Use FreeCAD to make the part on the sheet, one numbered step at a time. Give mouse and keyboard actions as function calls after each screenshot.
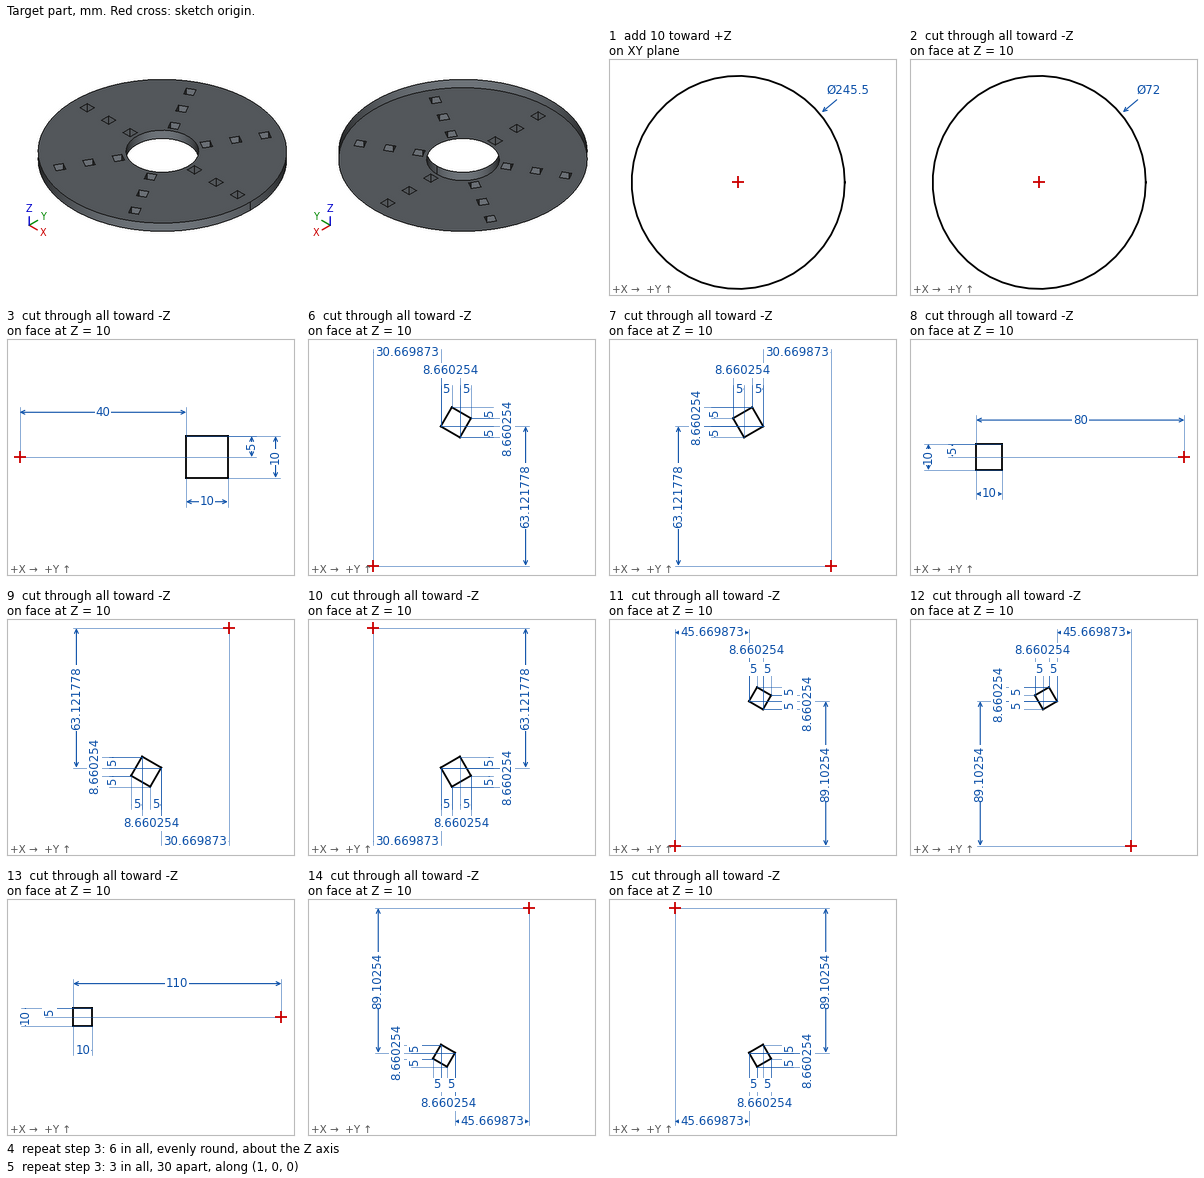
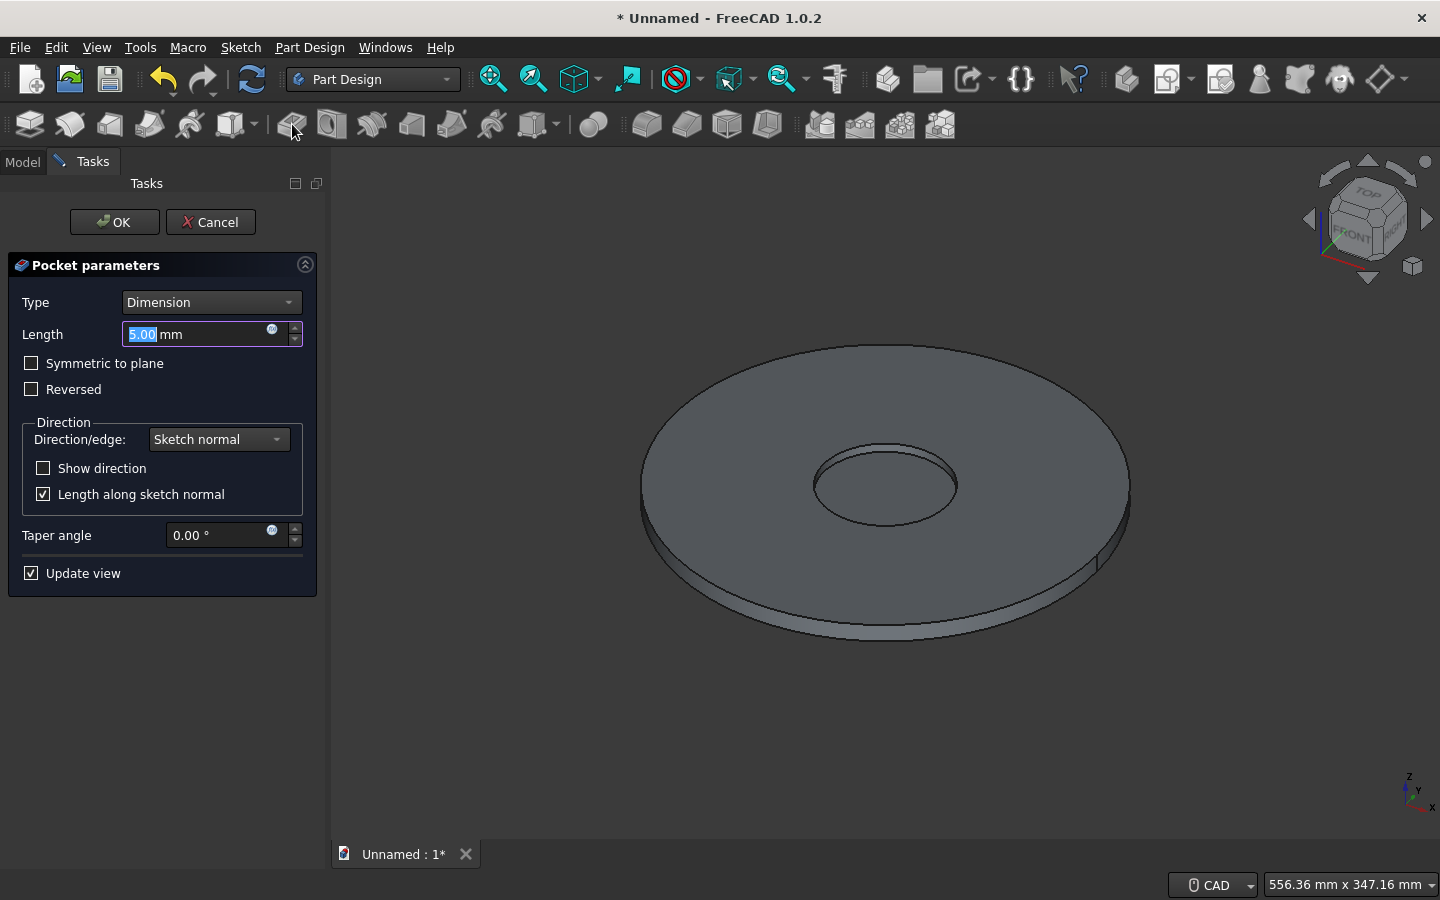
click(212, 302)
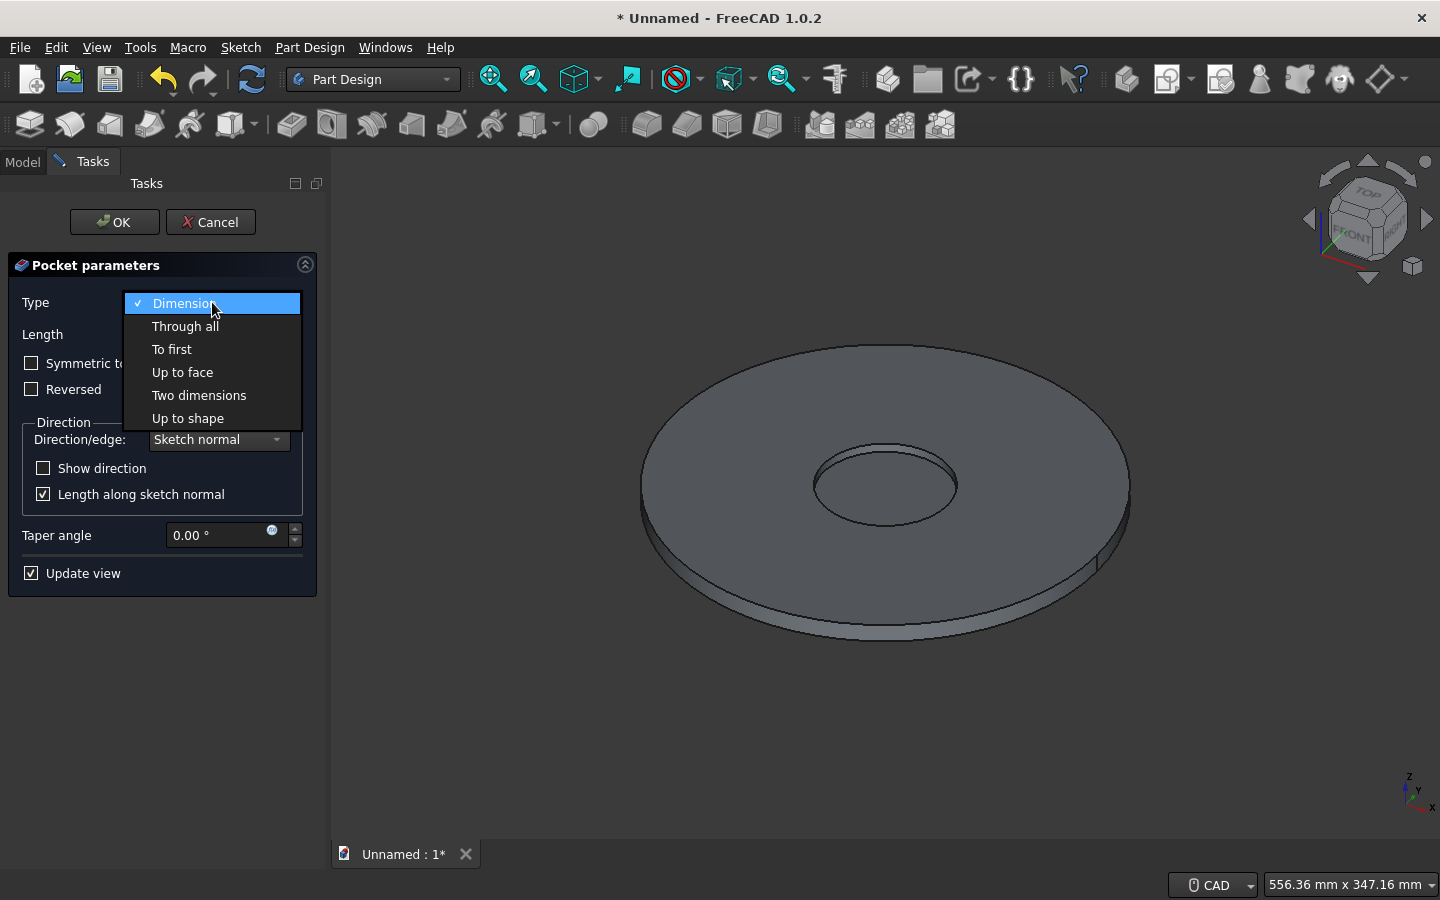
click(212, 326)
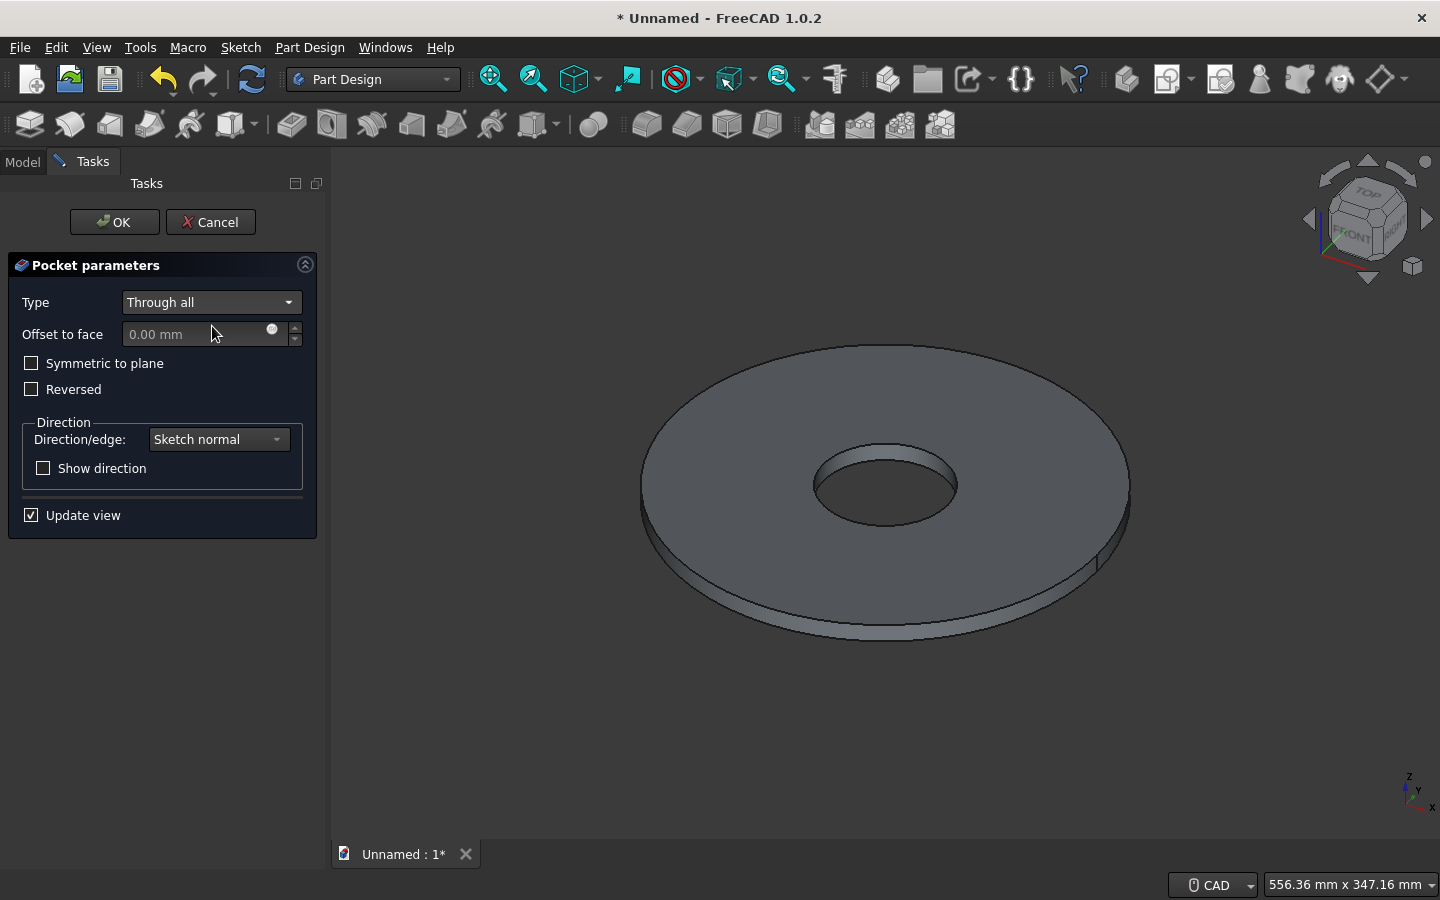
click(115, 222)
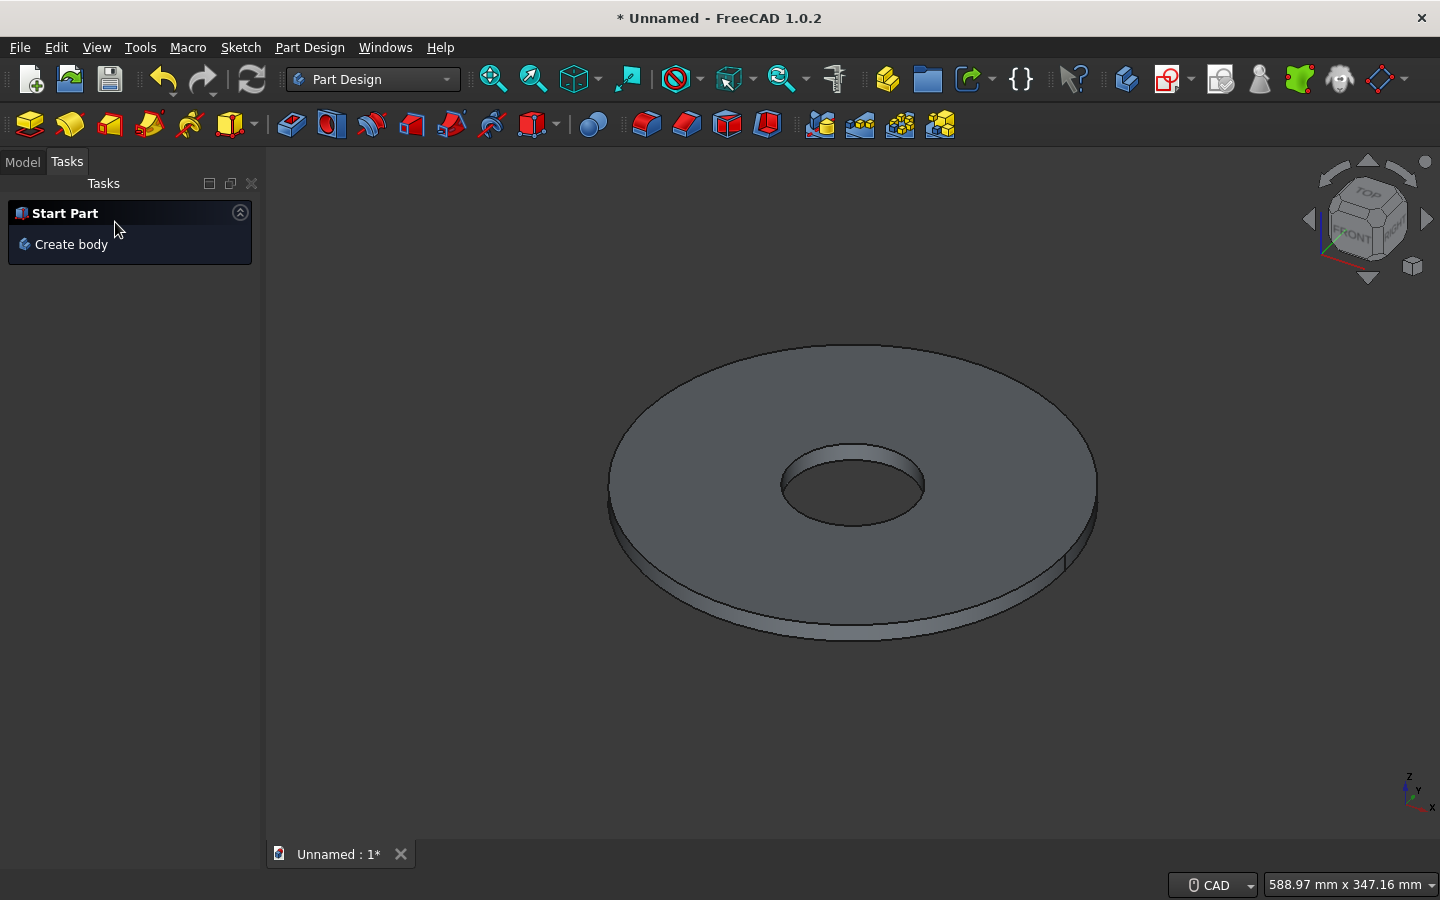
click(1009, 489)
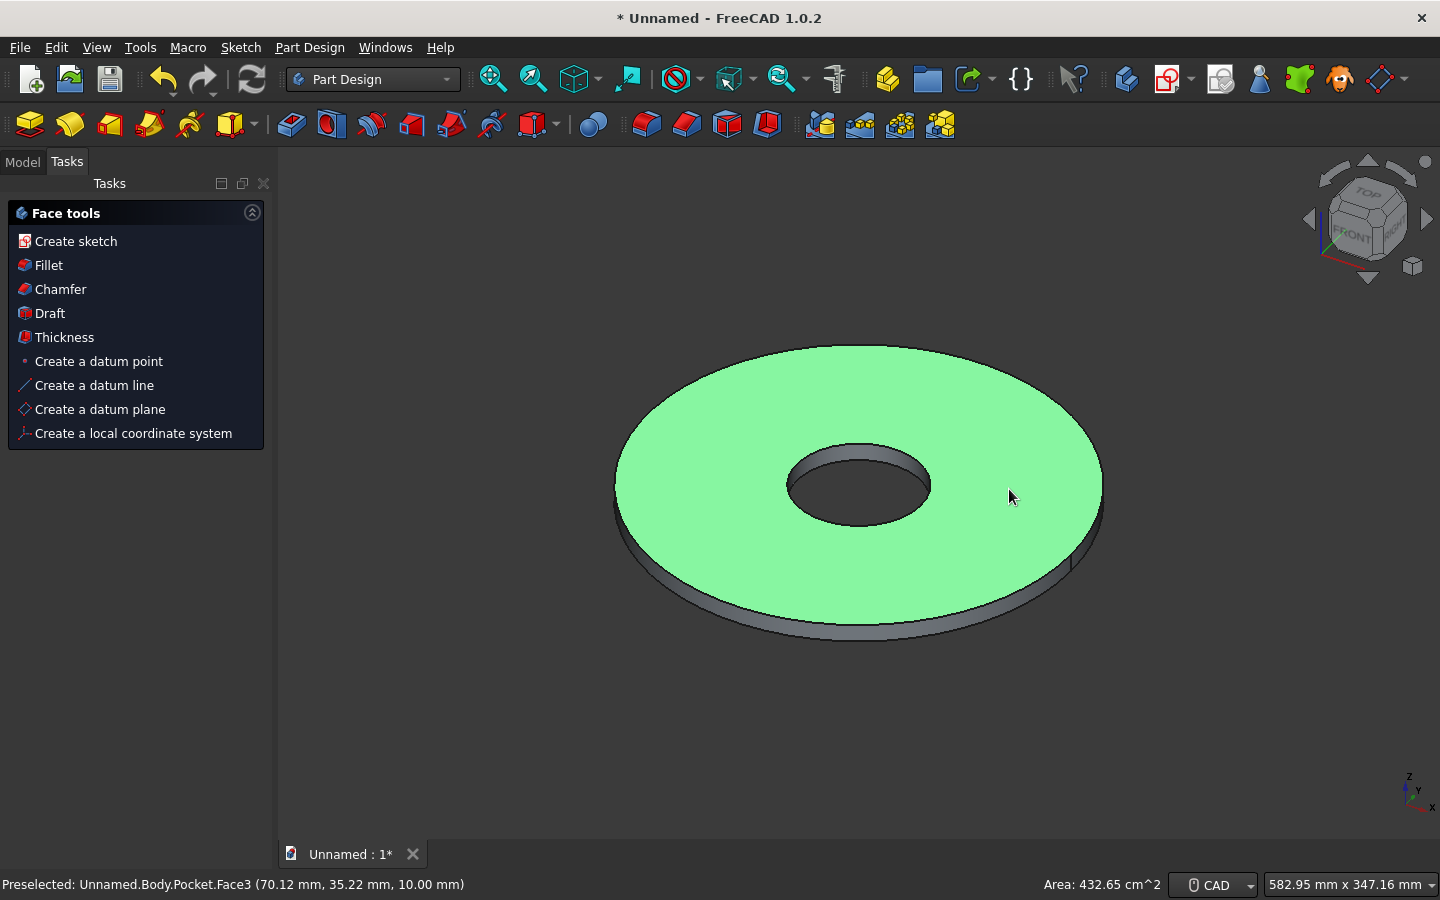
click(1168, 80)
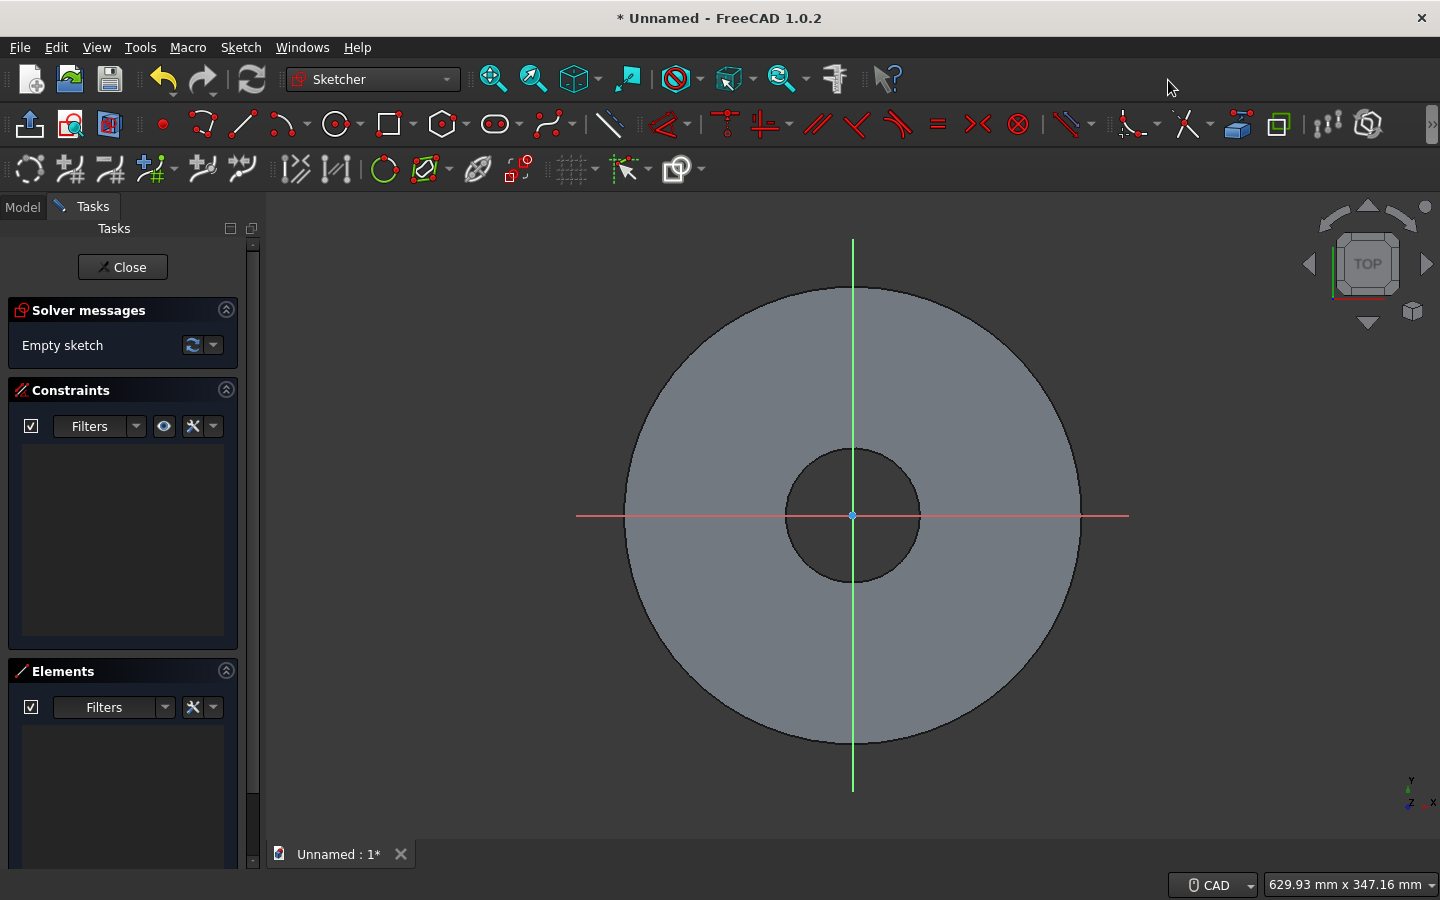
scroll(945, 516, up, 15)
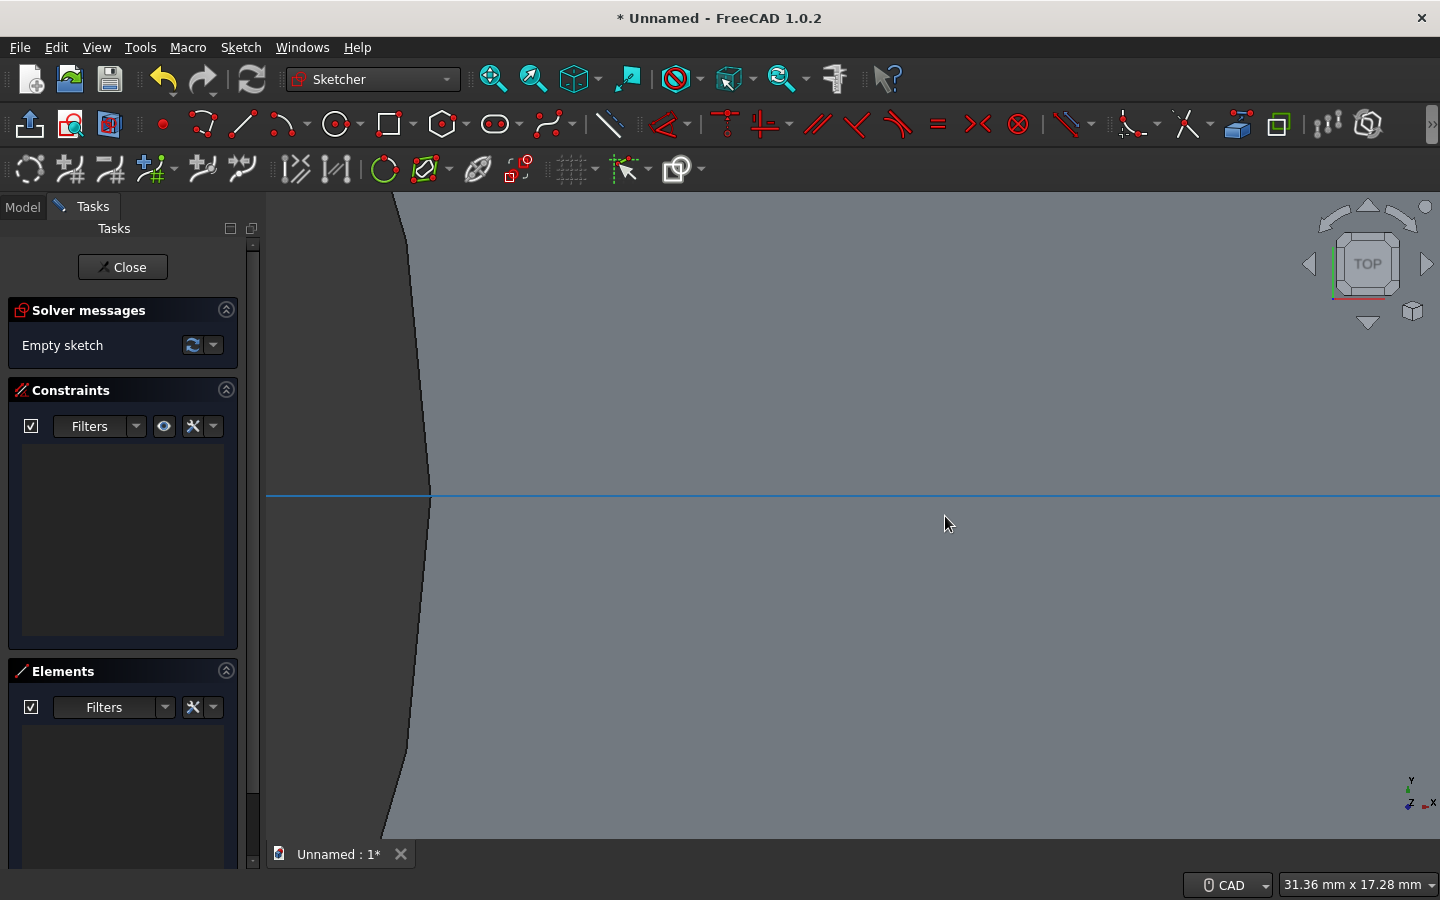
click(390, 124)